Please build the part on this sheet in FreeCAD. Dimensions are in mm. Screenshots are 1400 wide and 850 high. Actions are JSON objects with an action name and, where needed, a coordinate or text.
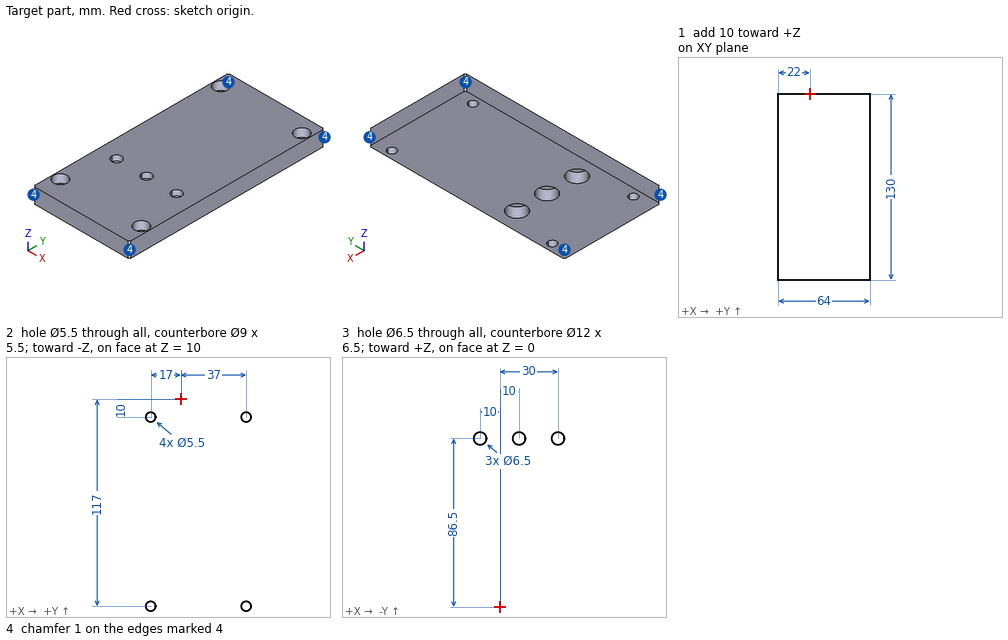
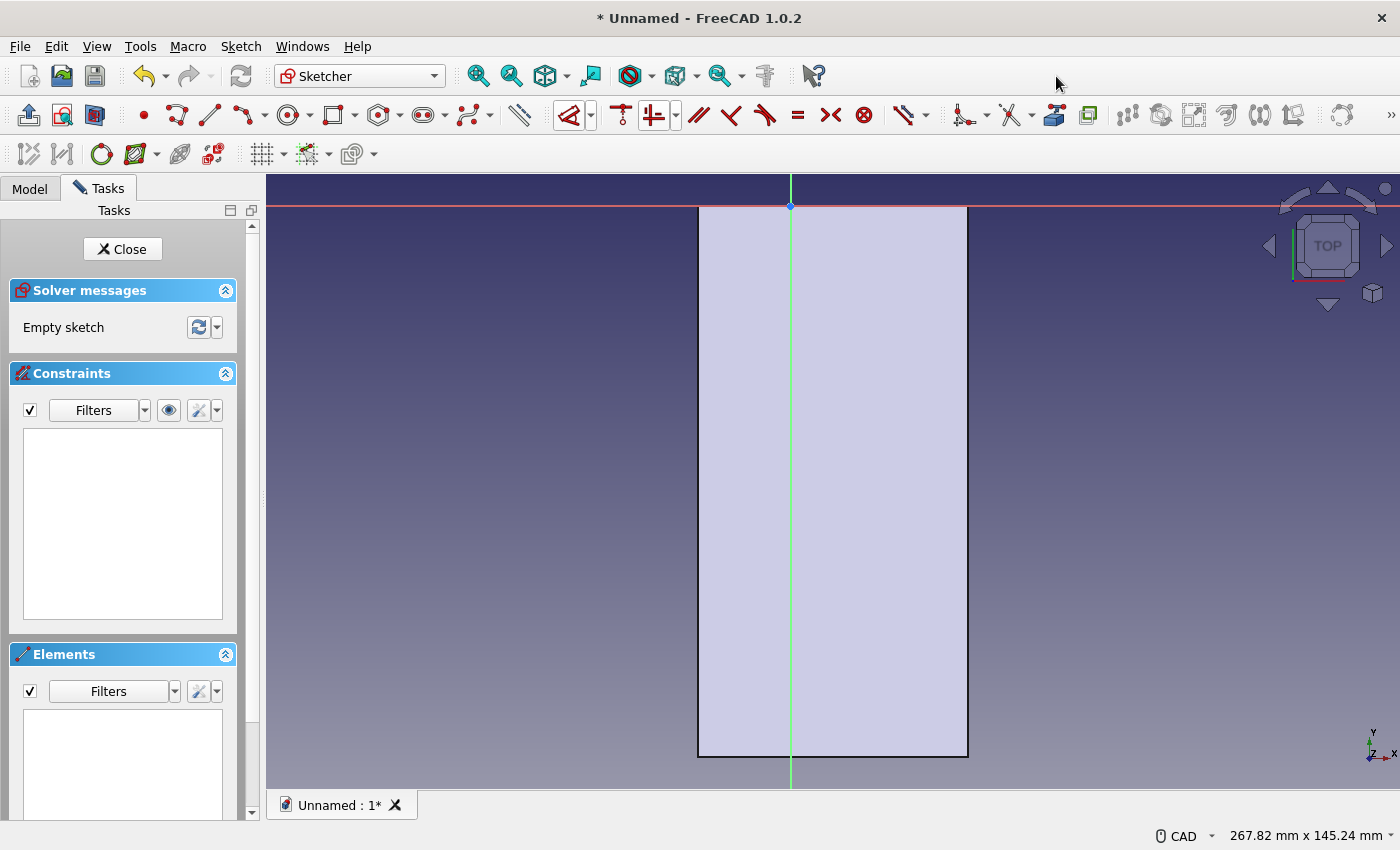
{"action": "scroll", "coordinate": [455, 580], "scroll_direction": "down", "scroll_amount": 1}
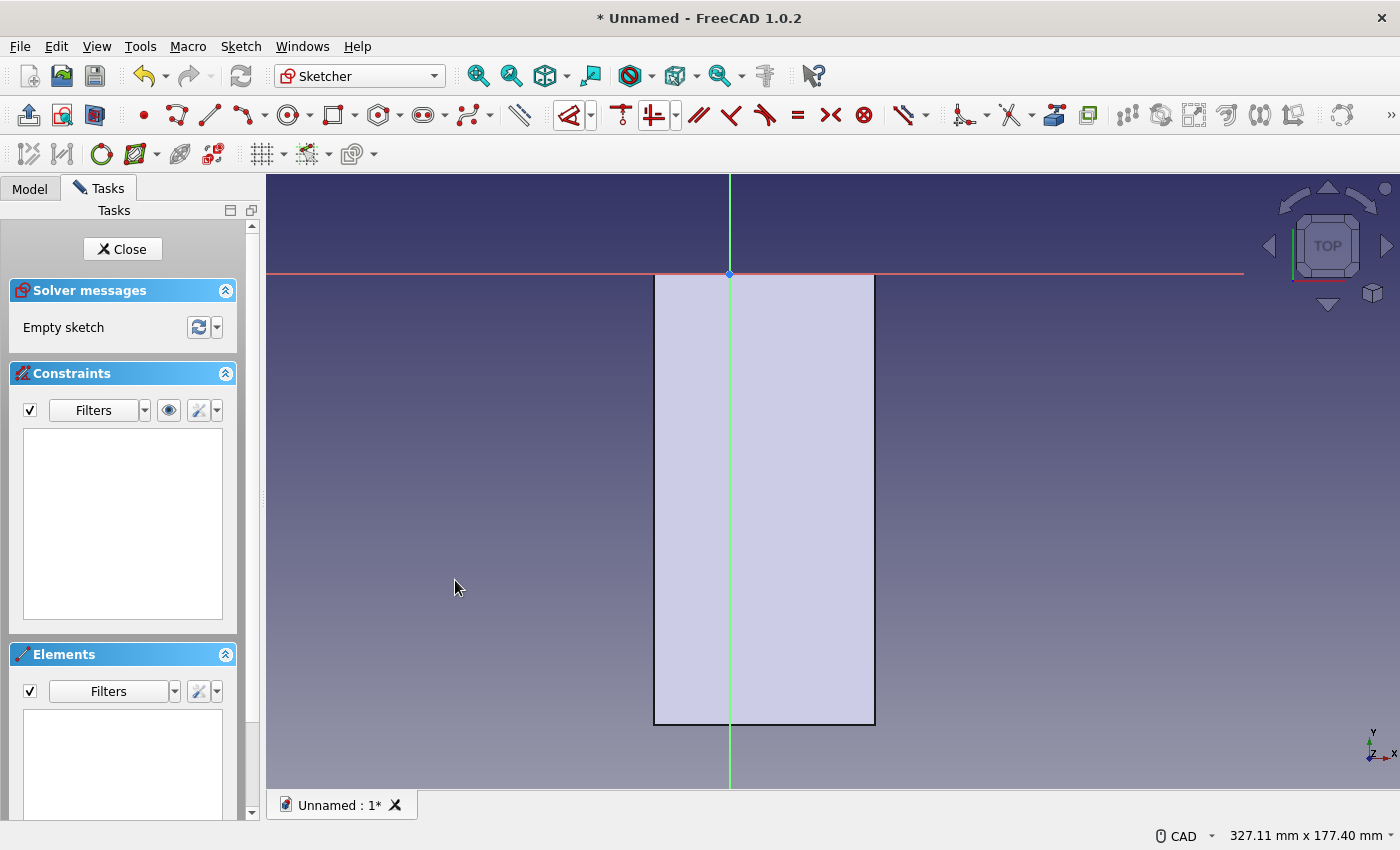
{"action": "key", "text": "g c"}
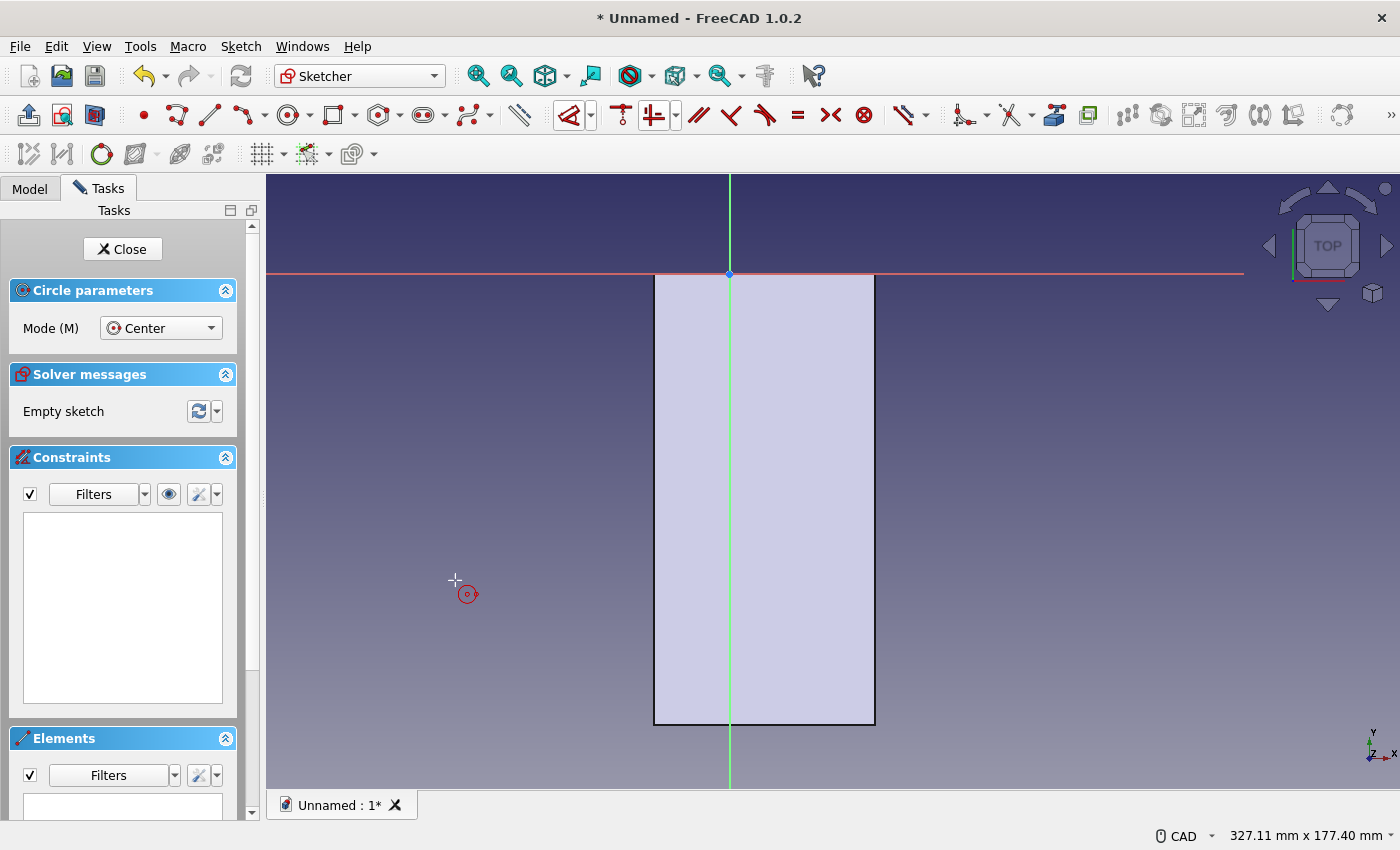
{"action": "scroll", "coordinate": [671, 309], "scroll_direction": "up", "scroll_amount": 5}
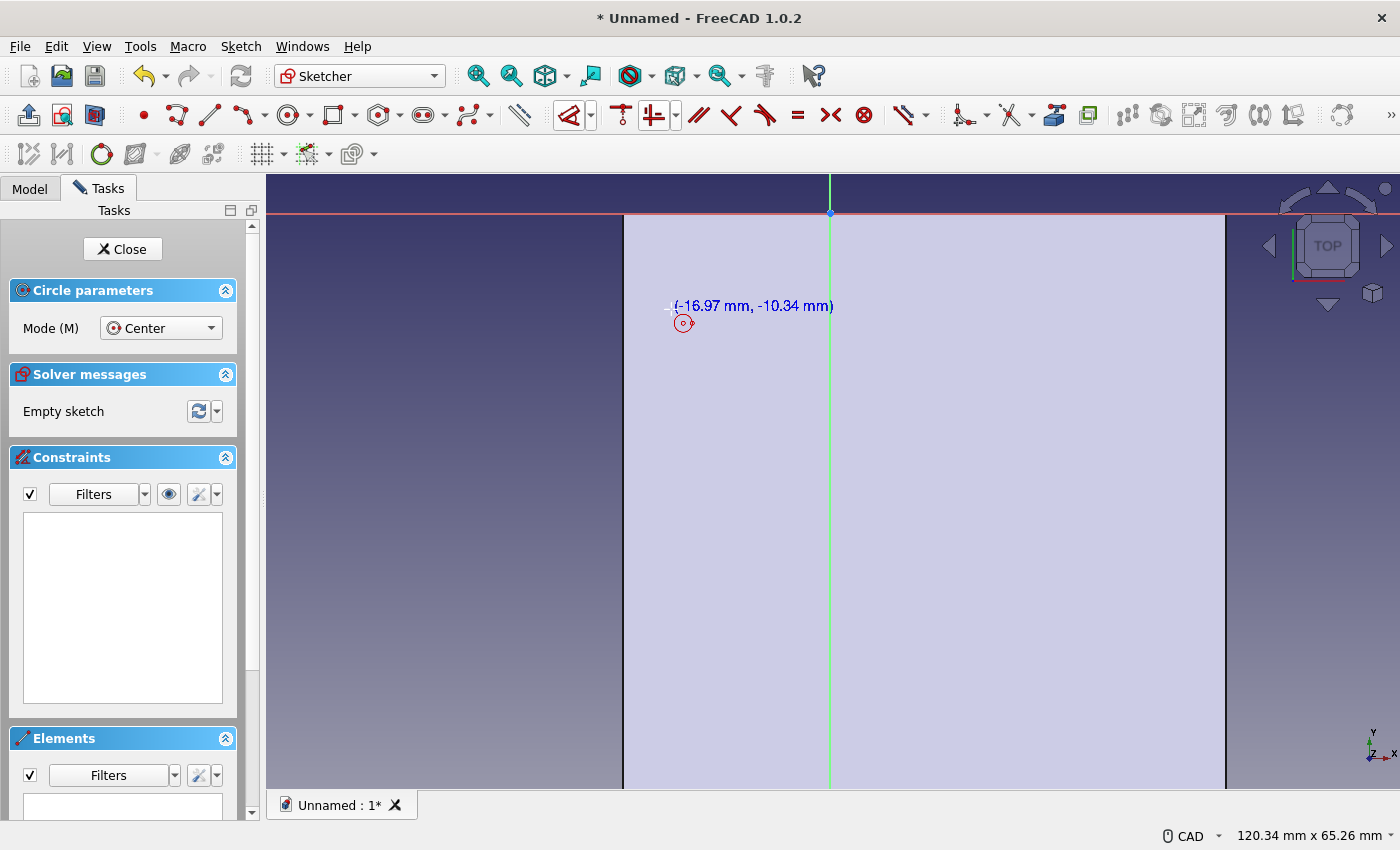
{"action": "left_click", "coordinate": [670, 308]}
{"action": "mouse_move", "coordinate": [688, 290]}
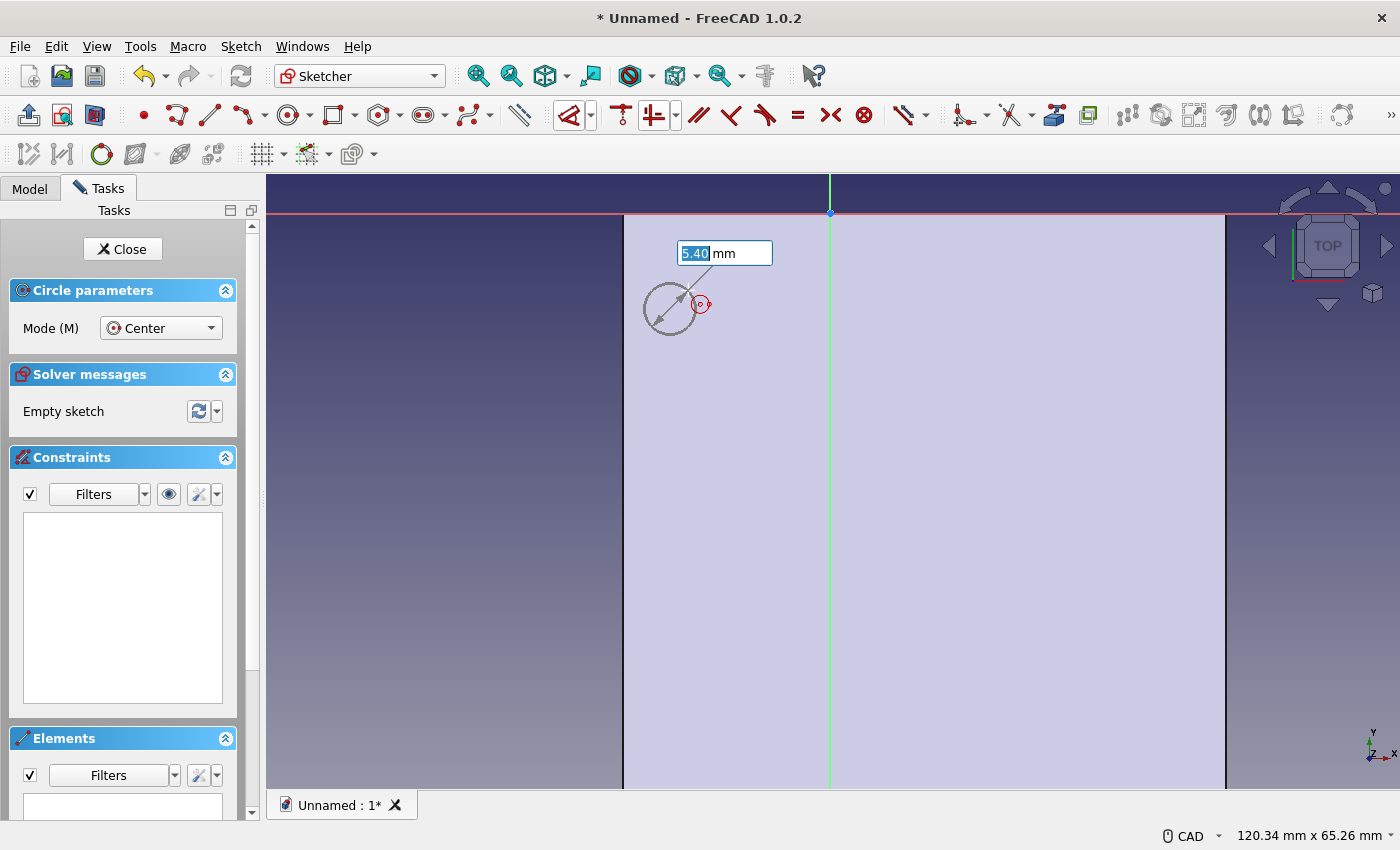
{"action": "type", "text": "5.5"}
{"action": "key", "text": "Return"}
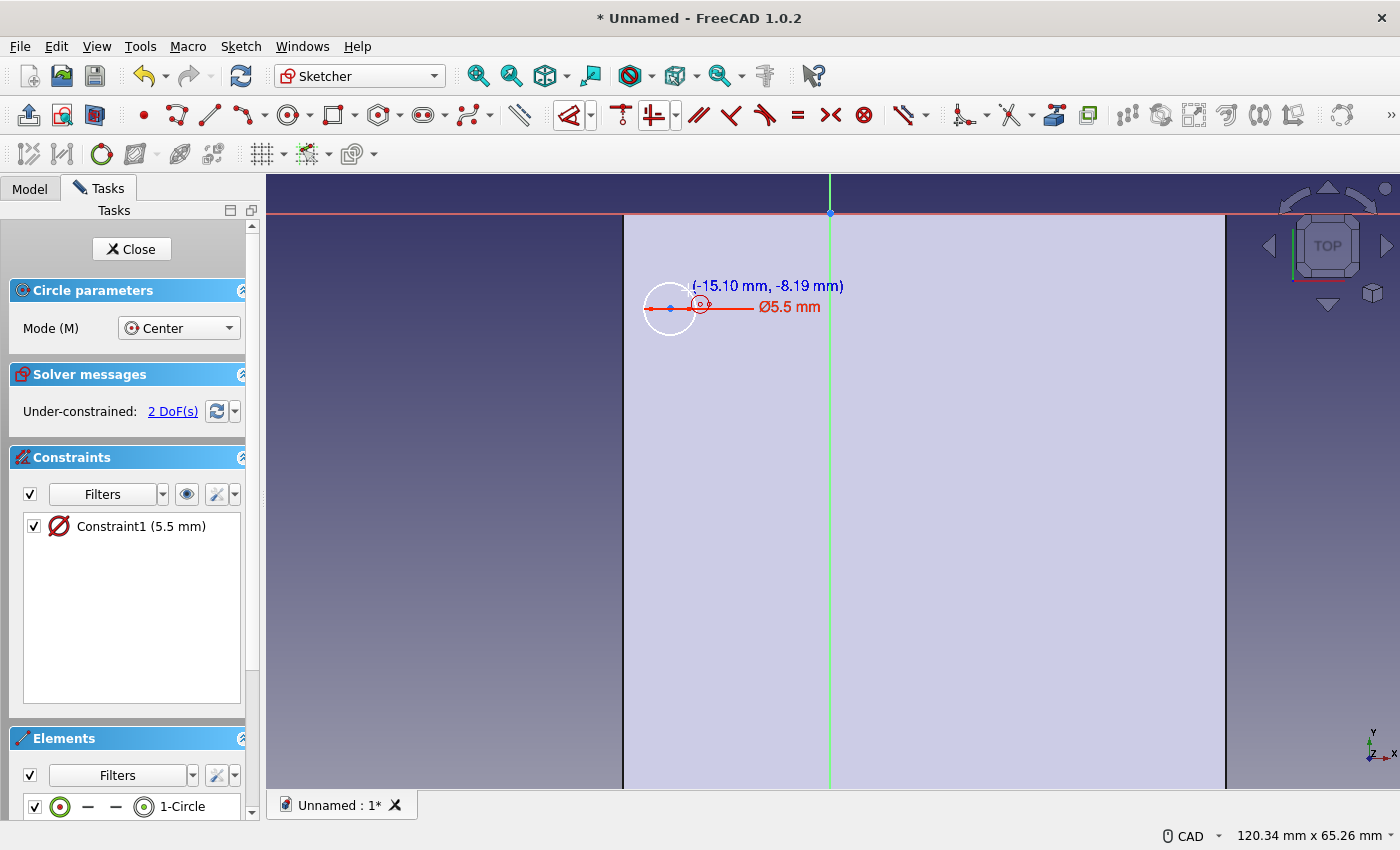
{"action": "left_click", "coordinate": [1179, 308]}
{"action": "mouse_move", "coordinate": [1197, 290]}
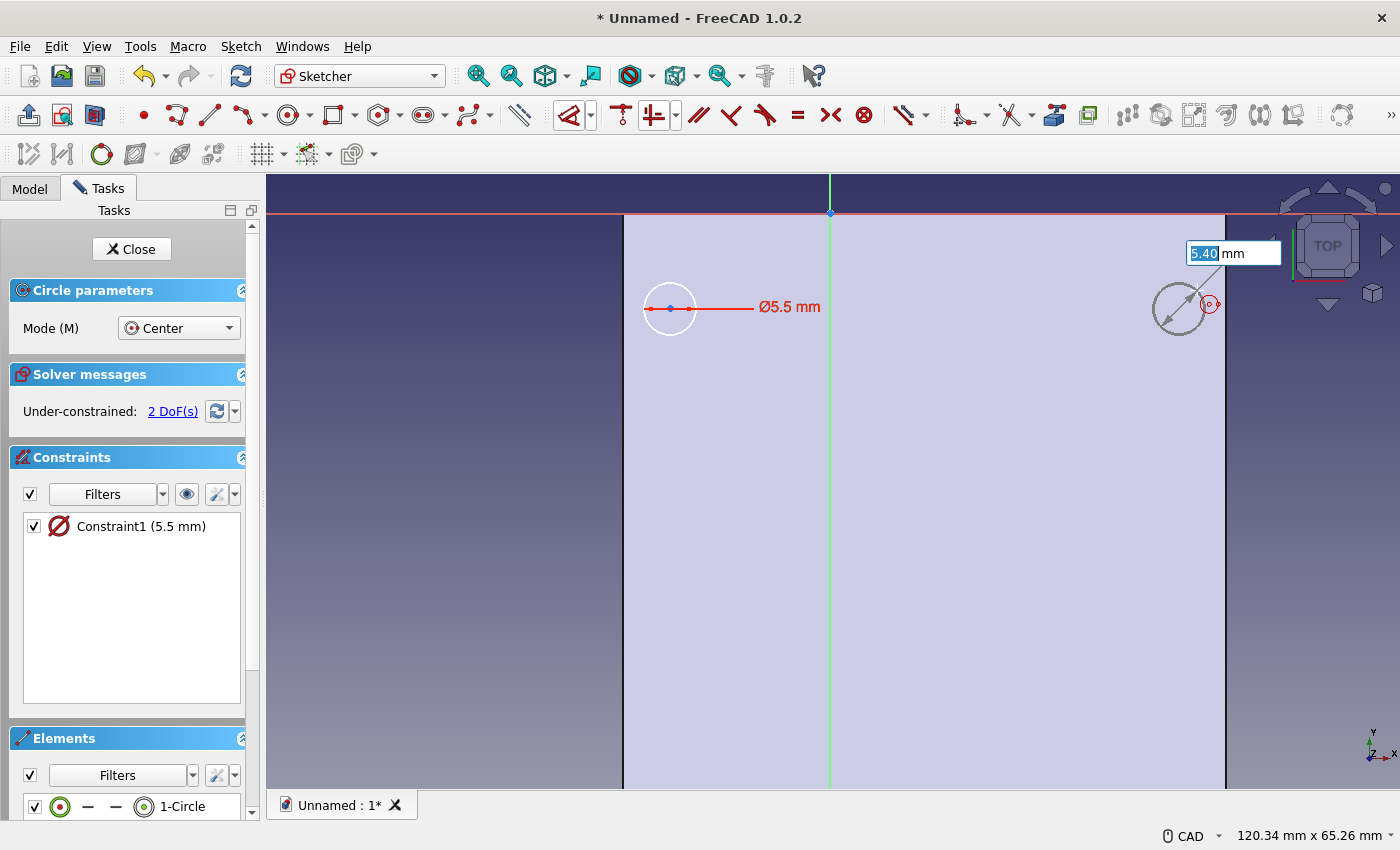
{"action": "type", "text": "5.5"}
{"action": "key", "text": "Return"}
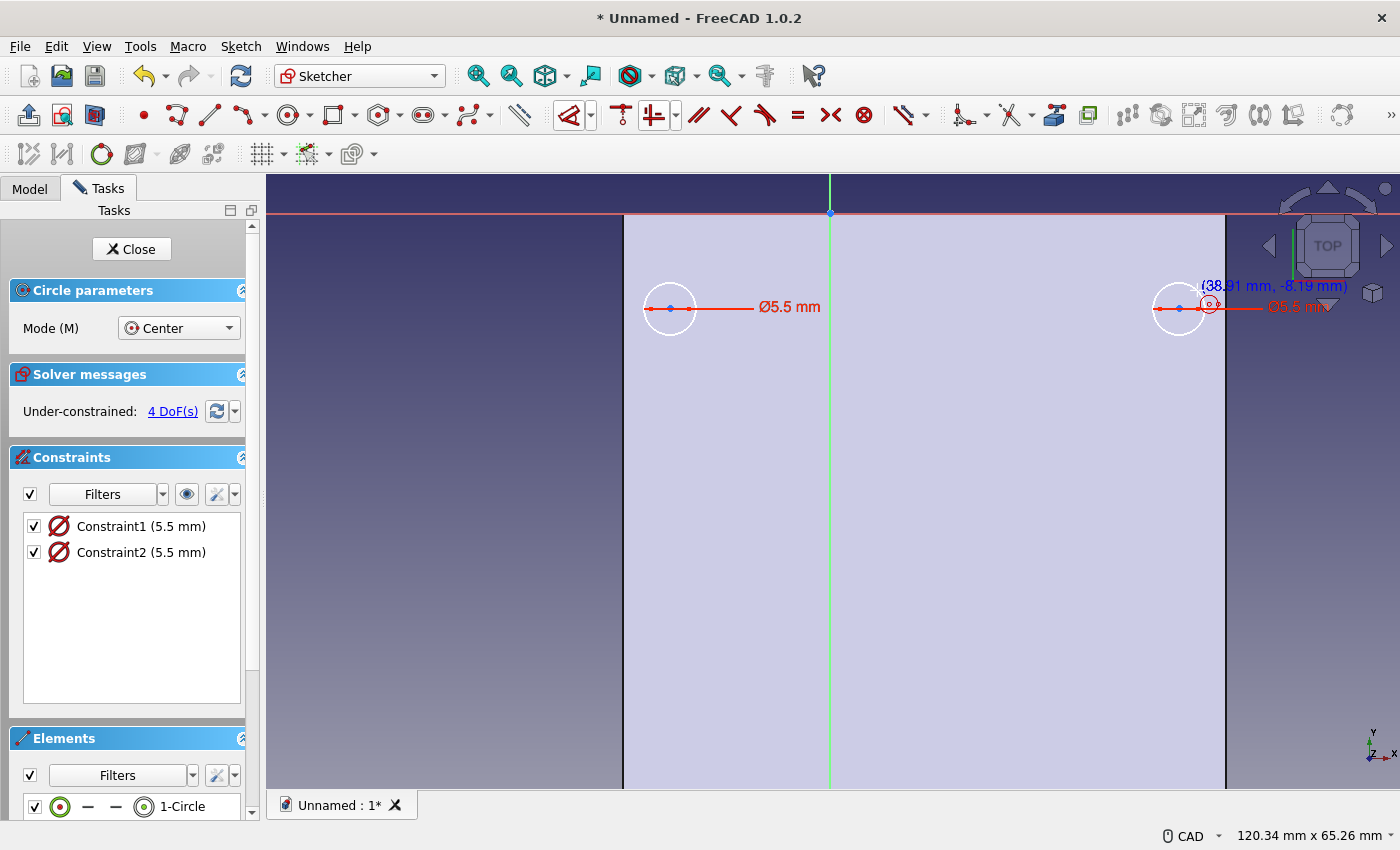
{"action": "scroll", "coordinate": [671, 309], "scroll_direction": "down", "scroll_amount": 5}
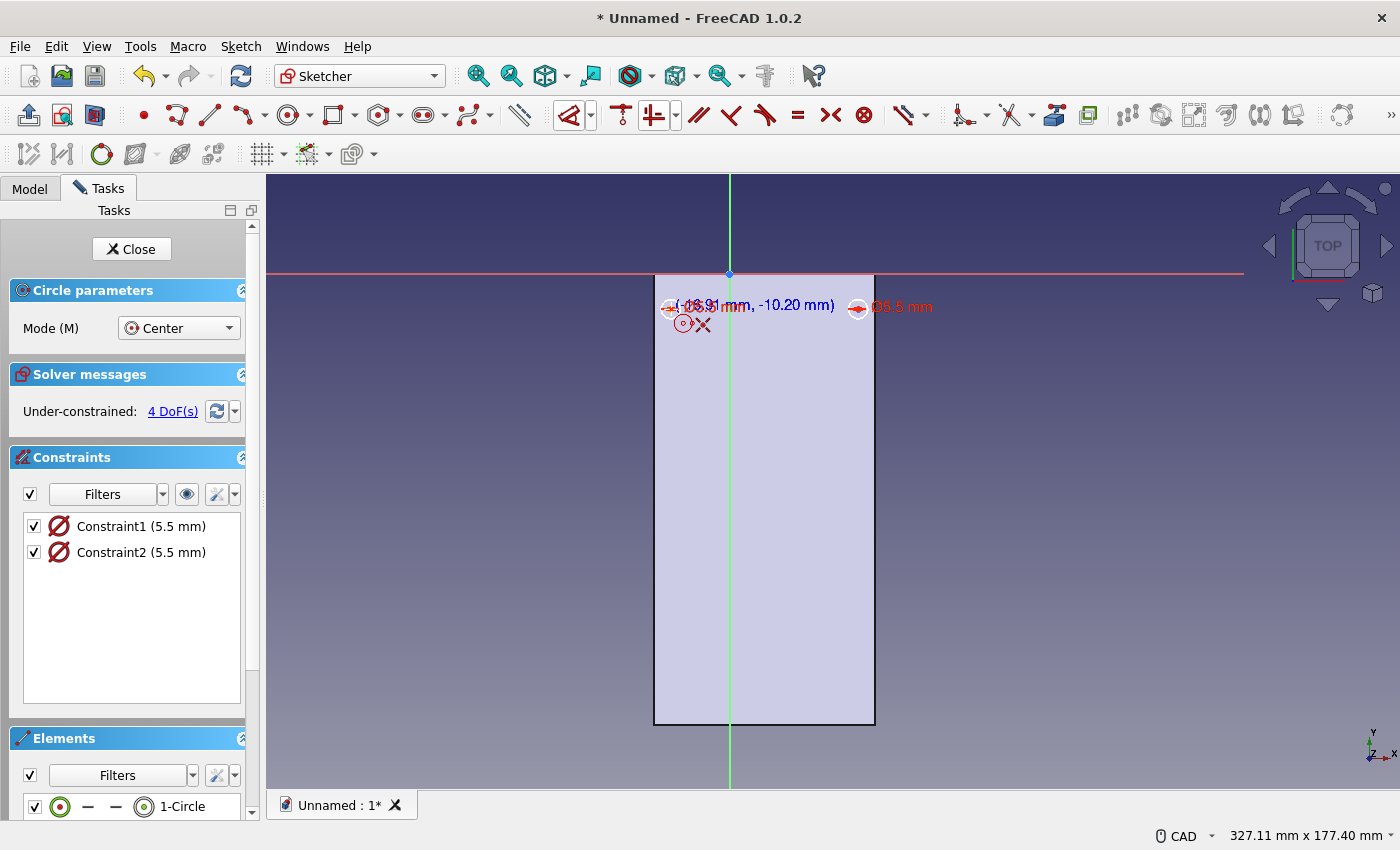
{"action": "scroll", "coordinate": [671, 680], "scroll_direction": "up", "scroll_amount": 5}